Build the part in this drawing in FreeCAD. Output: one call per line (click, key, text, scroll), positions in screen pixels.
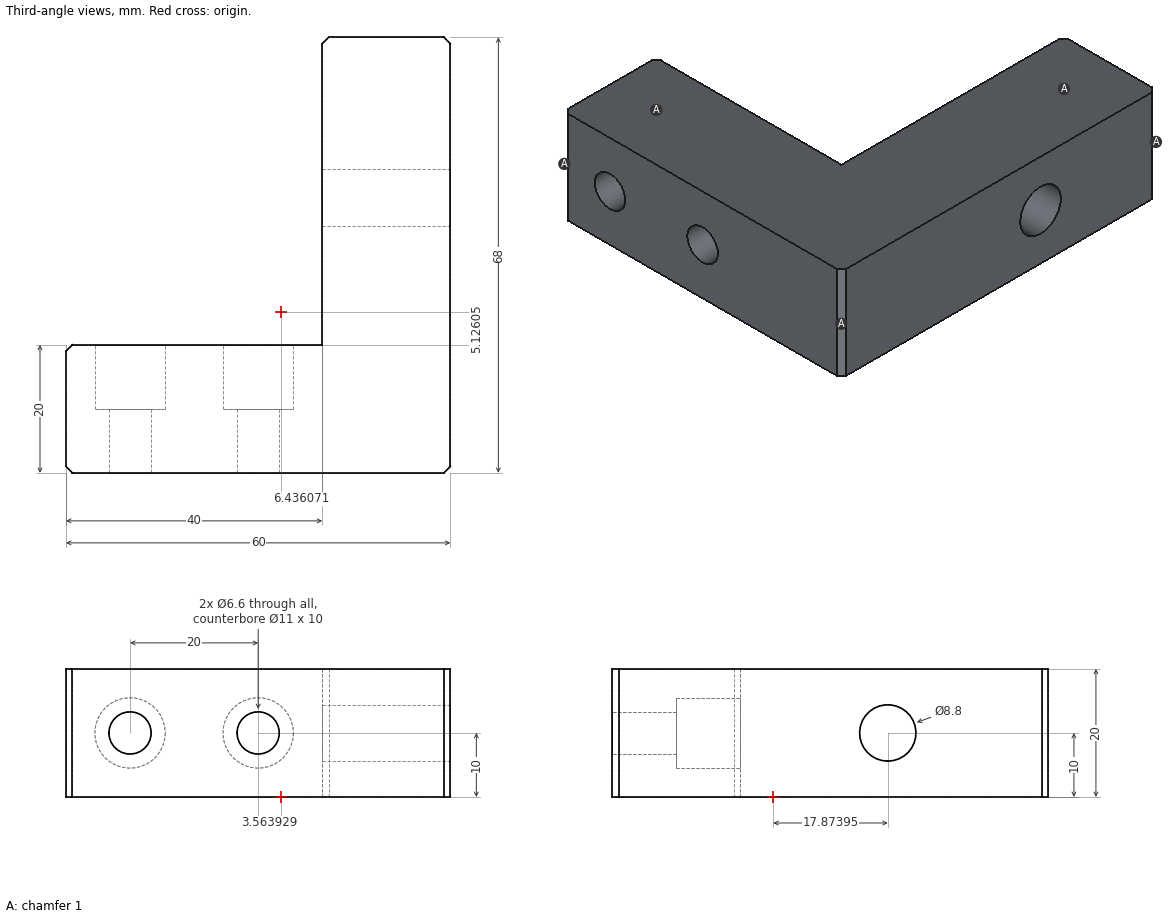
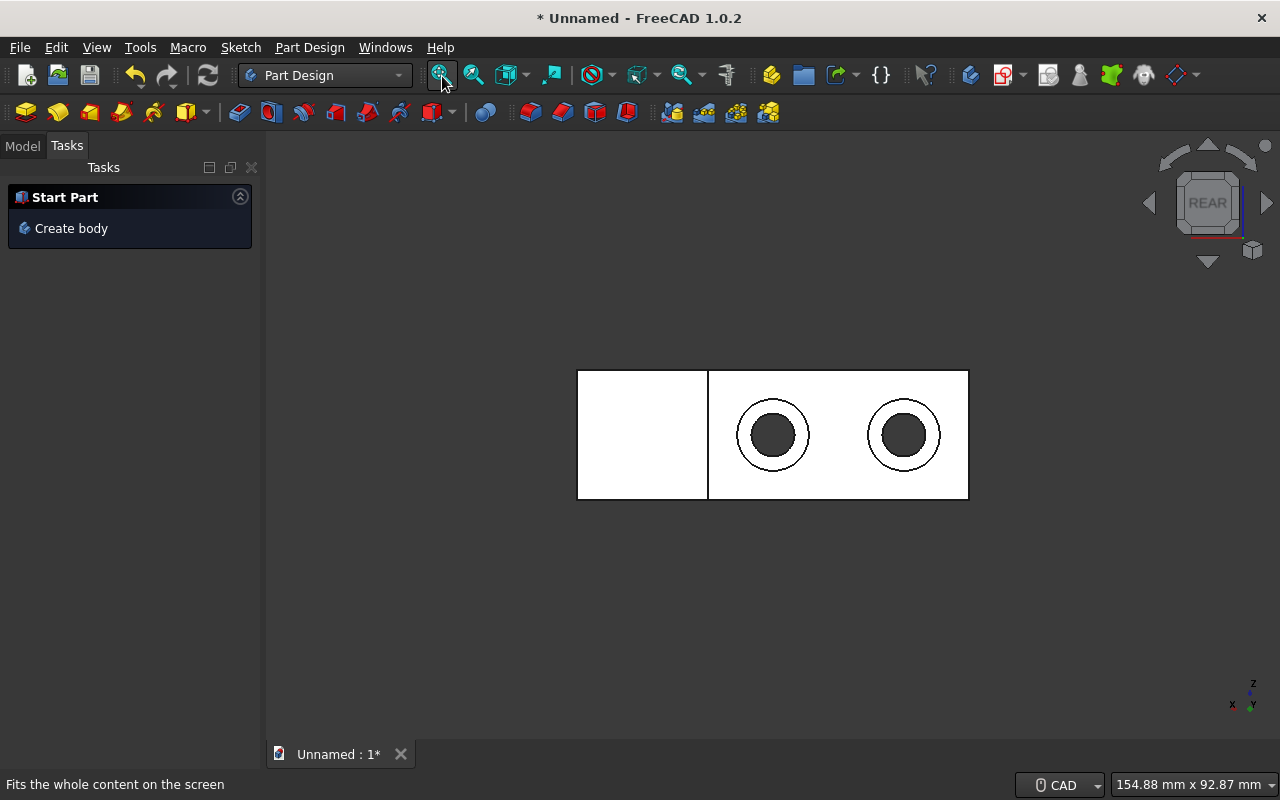
click(969, 434)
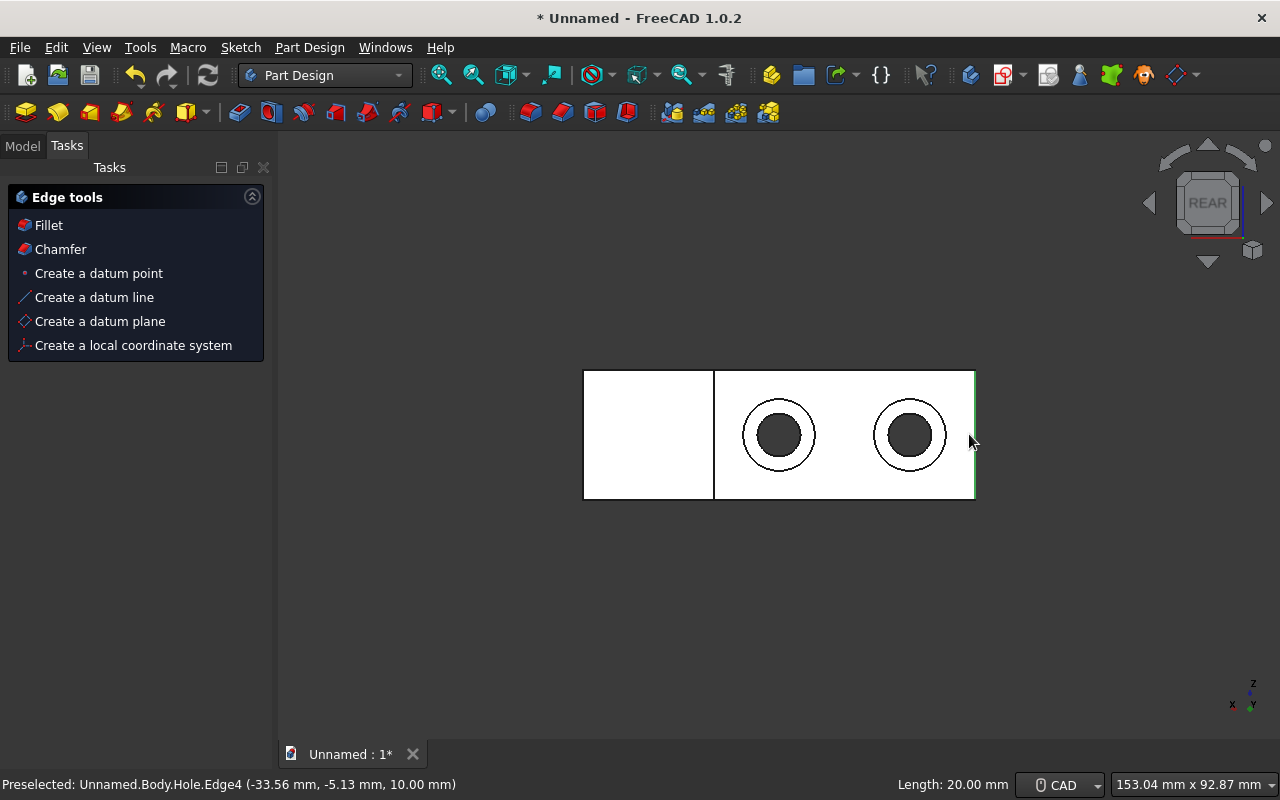
click(714, 434, ctrl)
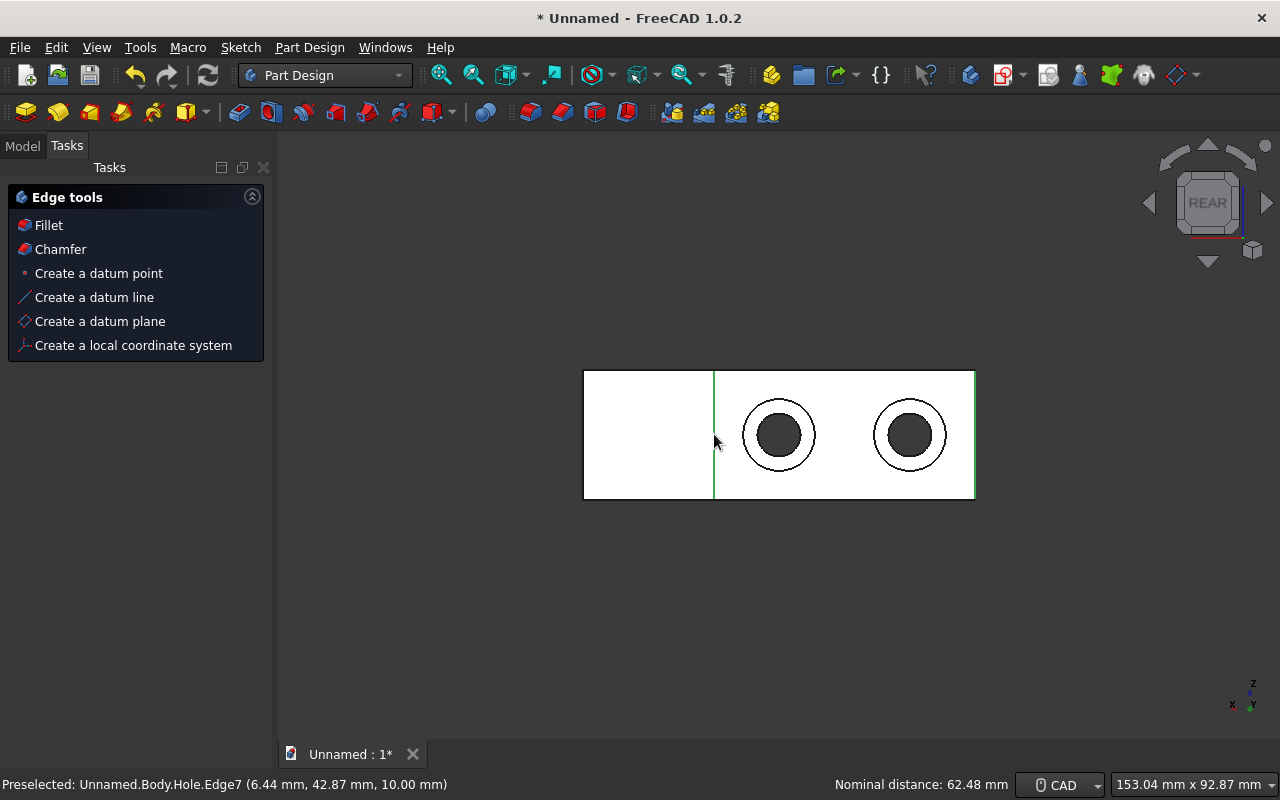
key(0)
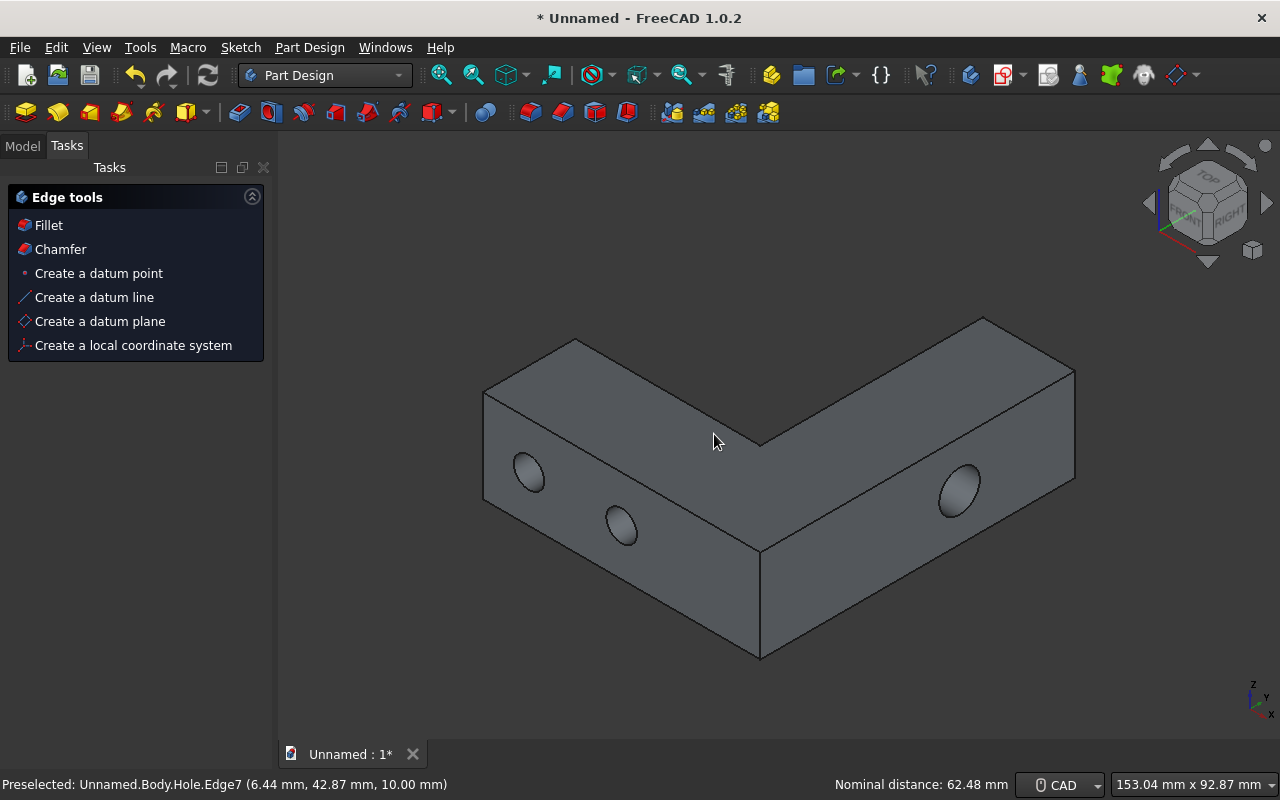
click(760, 605, ctrl)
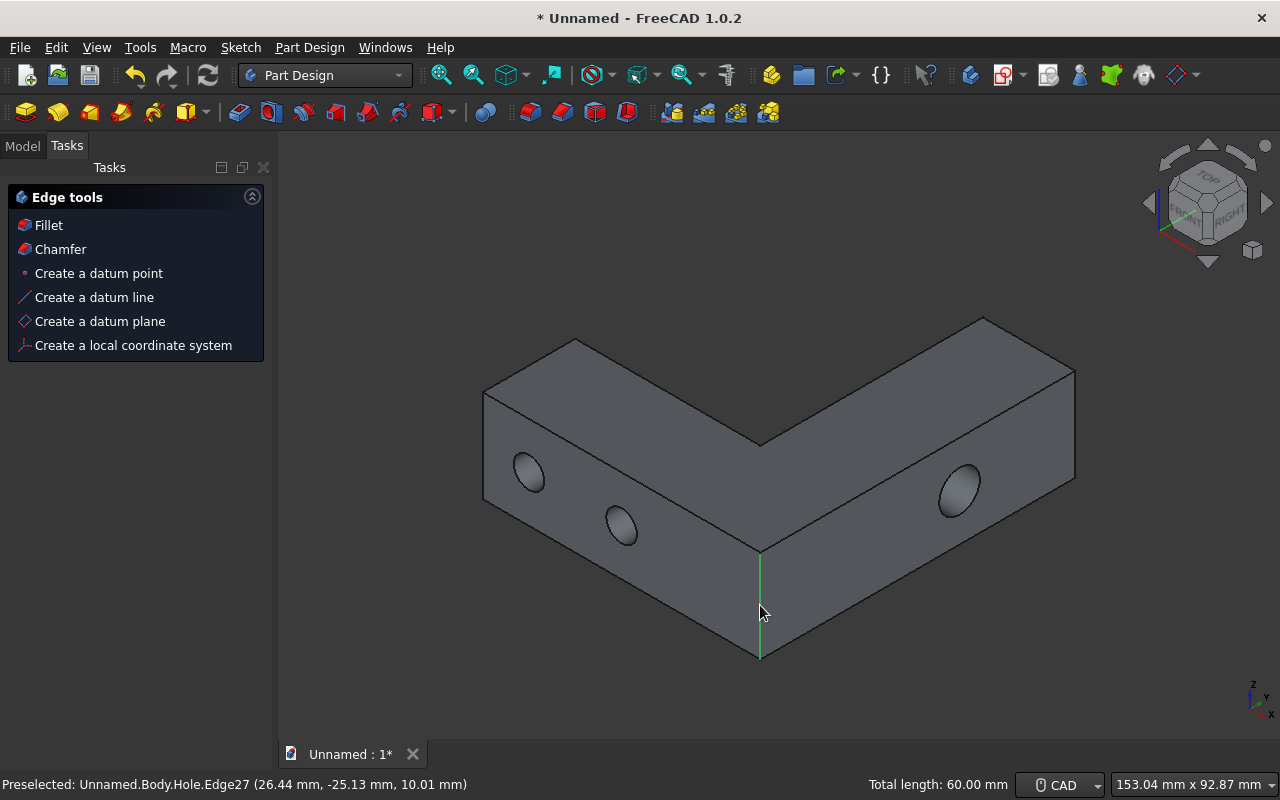
key(2)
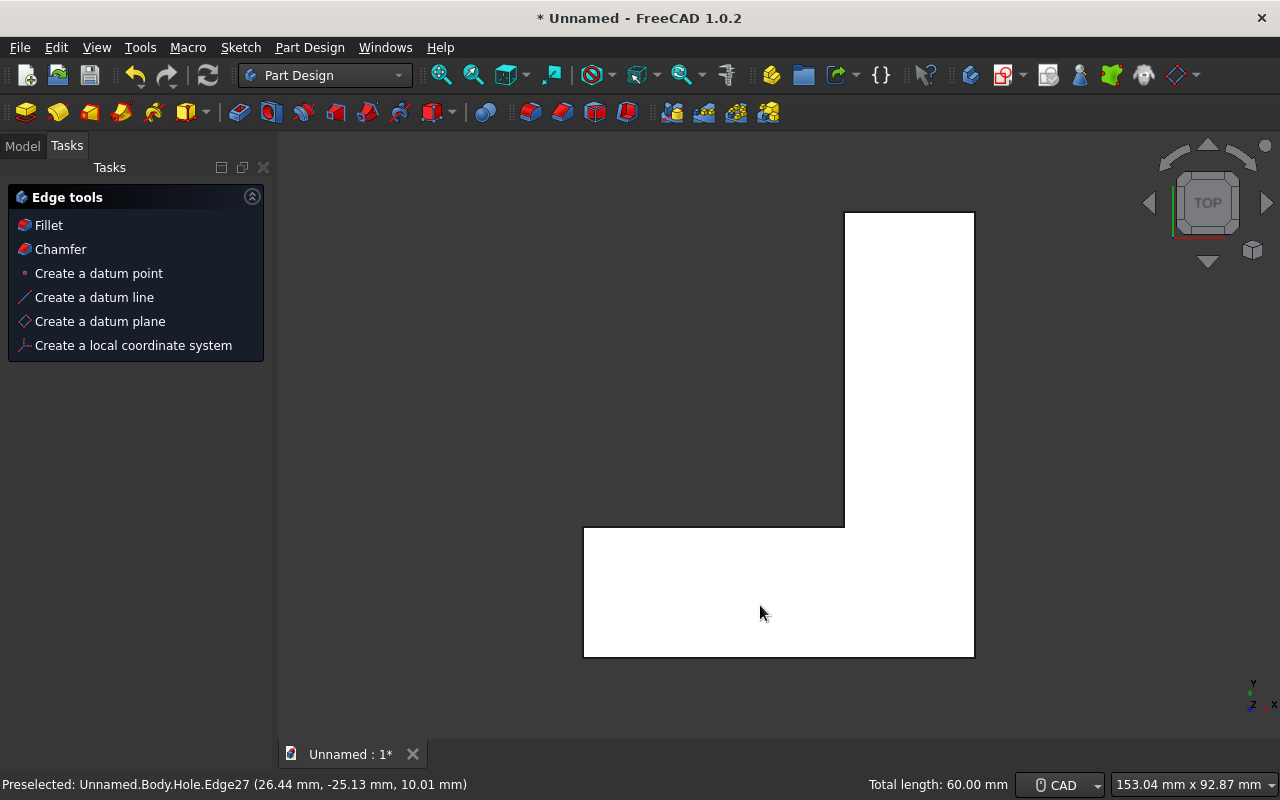
key(1)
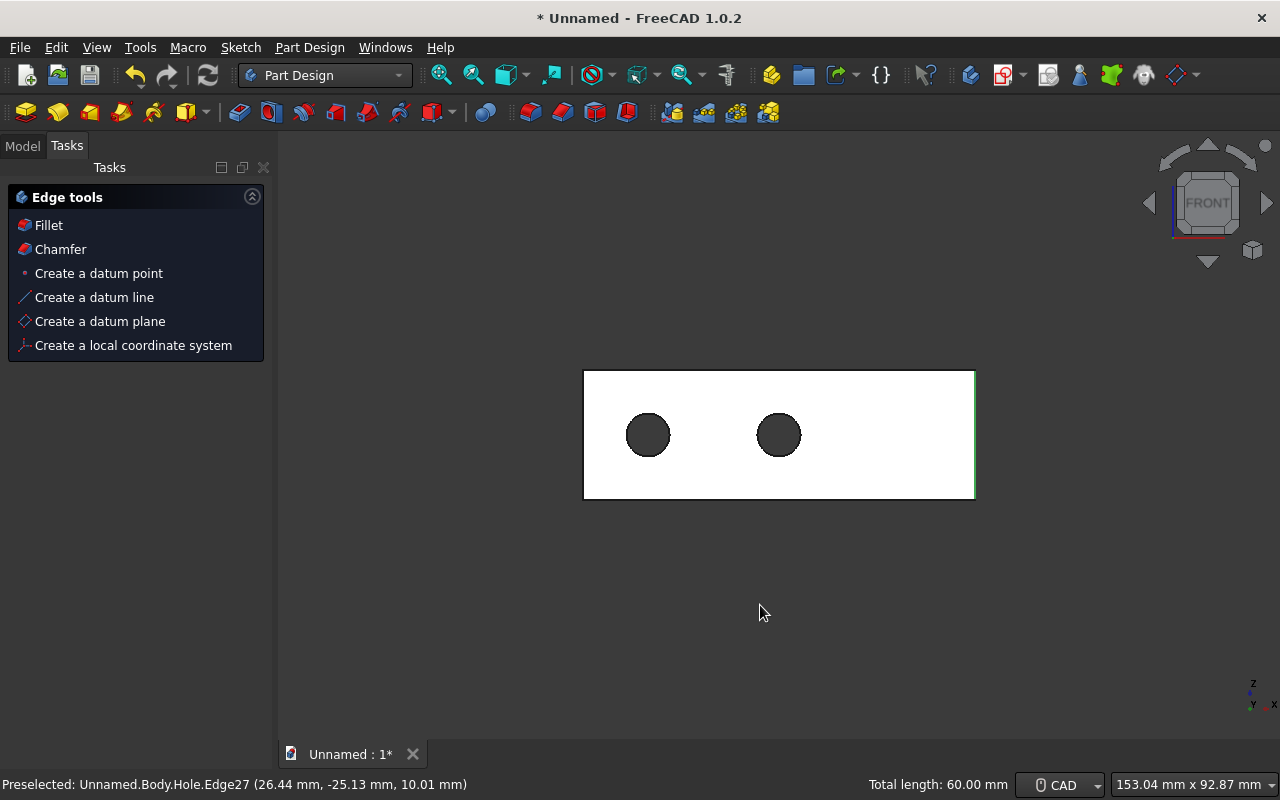
key(v)
key(f)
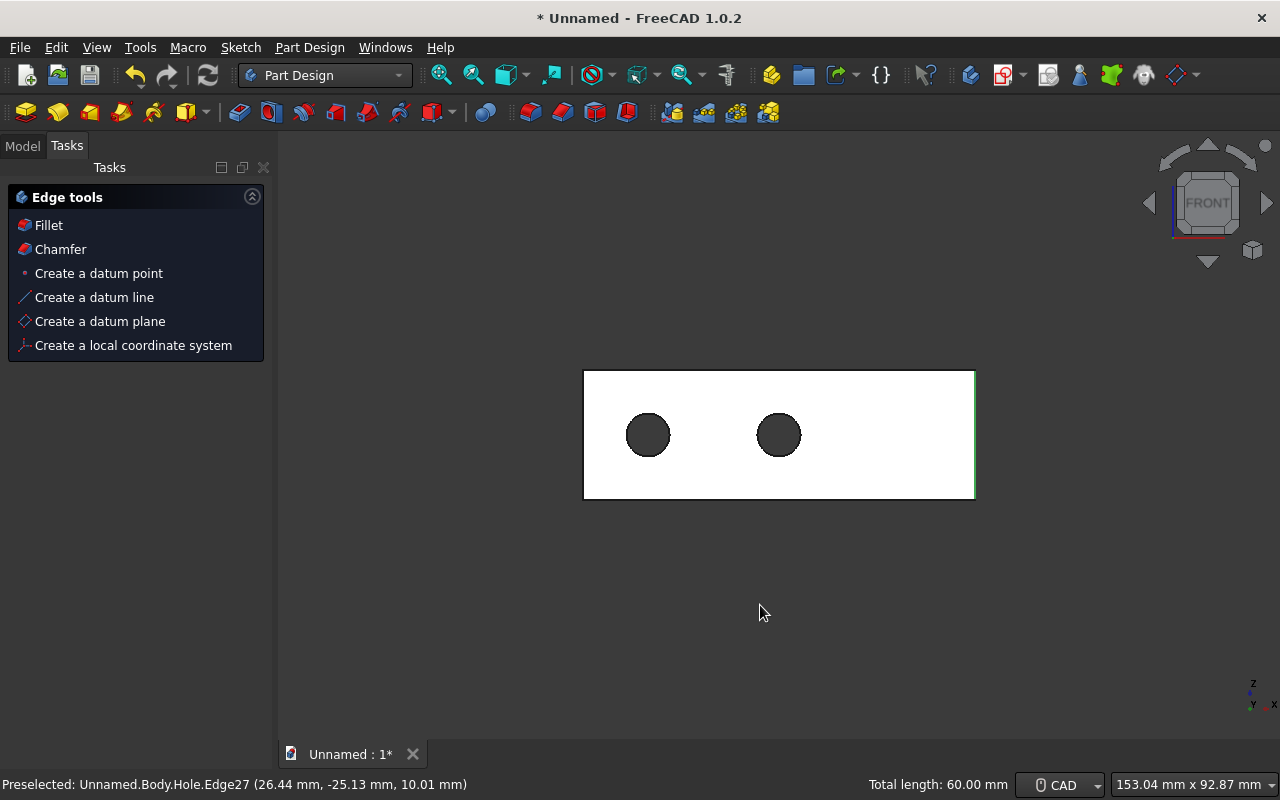
click(583, 434, ctrl)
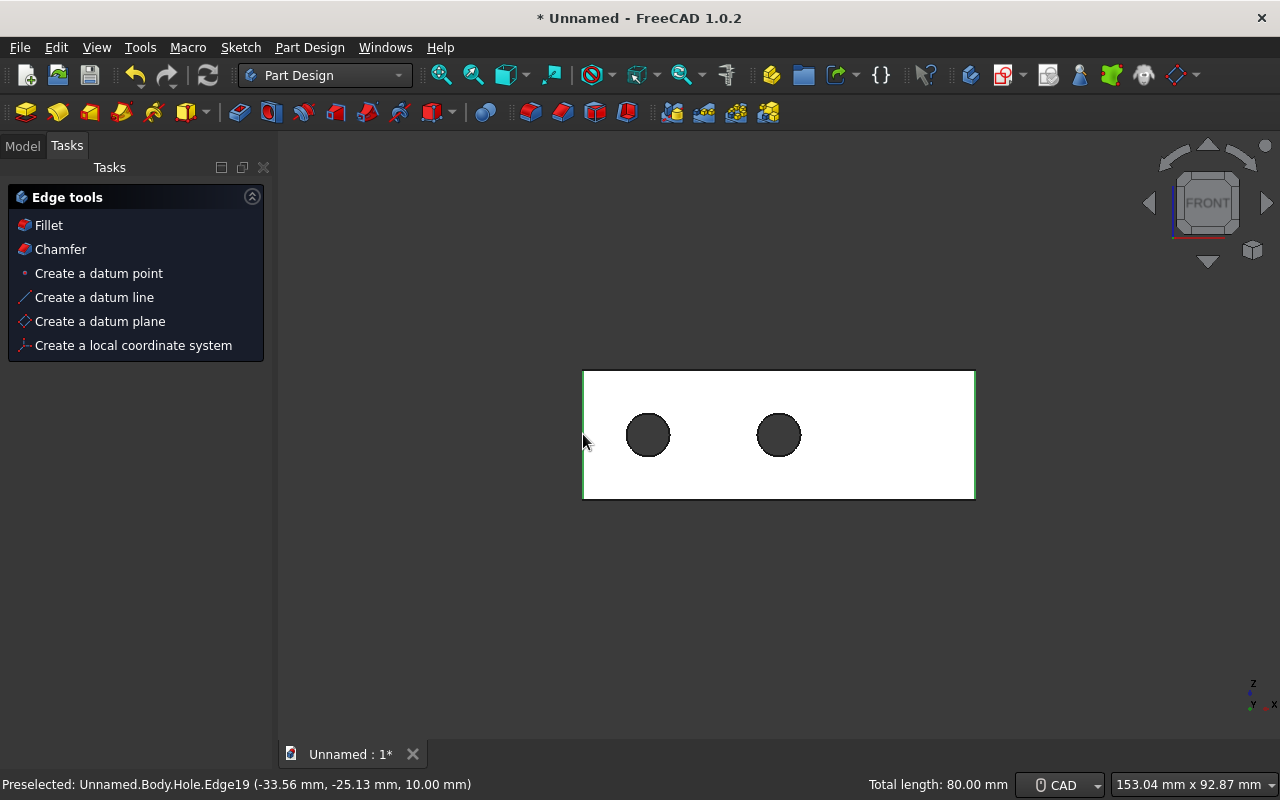
key(3)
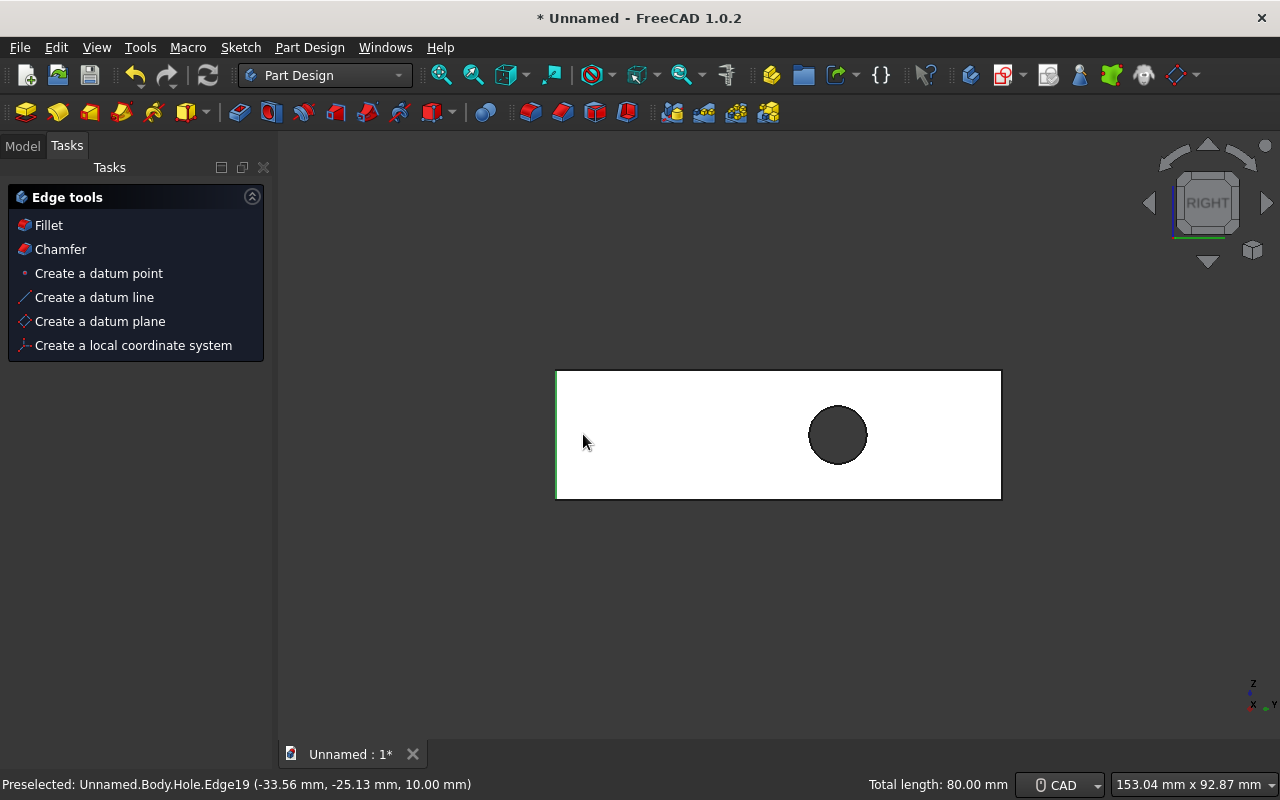
click(442, 76)